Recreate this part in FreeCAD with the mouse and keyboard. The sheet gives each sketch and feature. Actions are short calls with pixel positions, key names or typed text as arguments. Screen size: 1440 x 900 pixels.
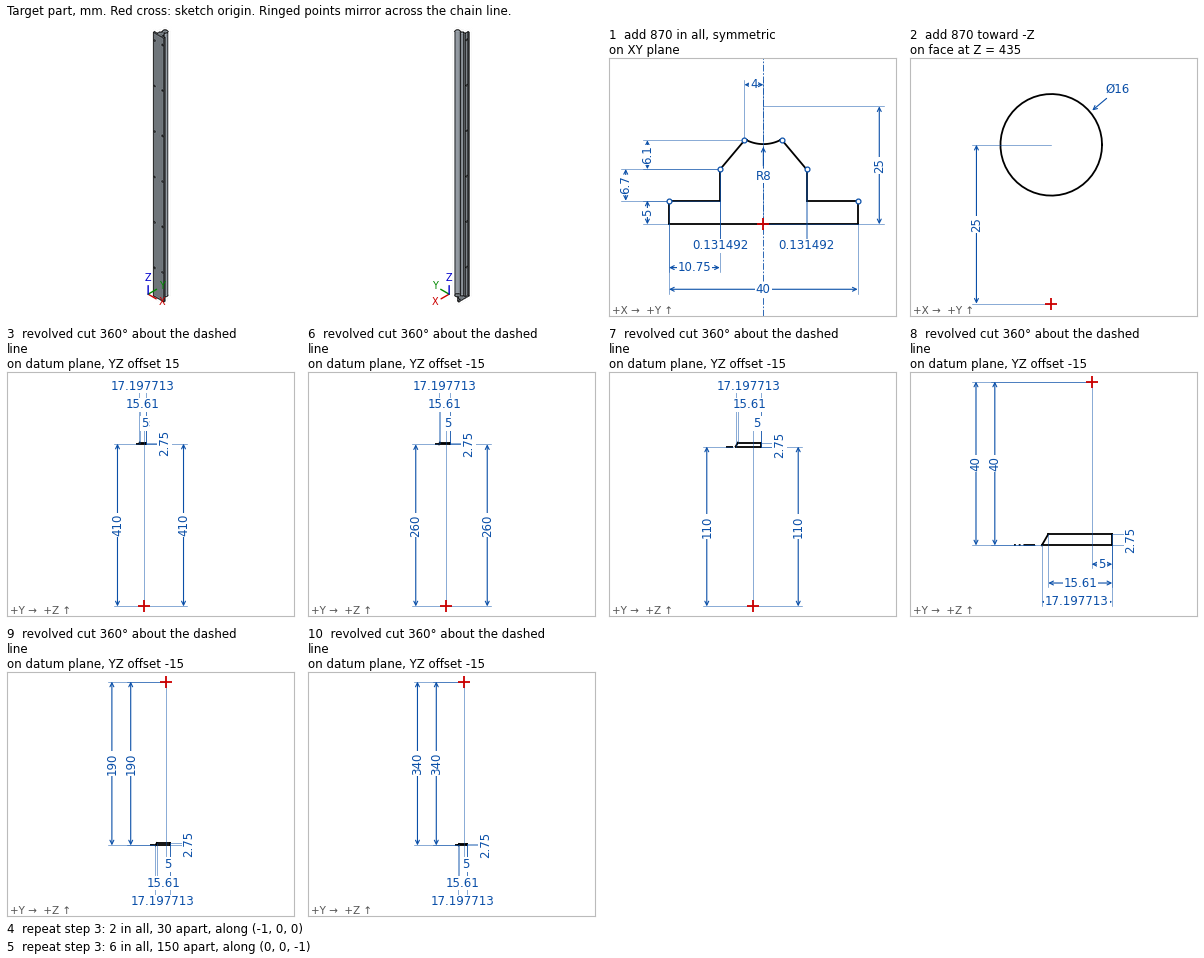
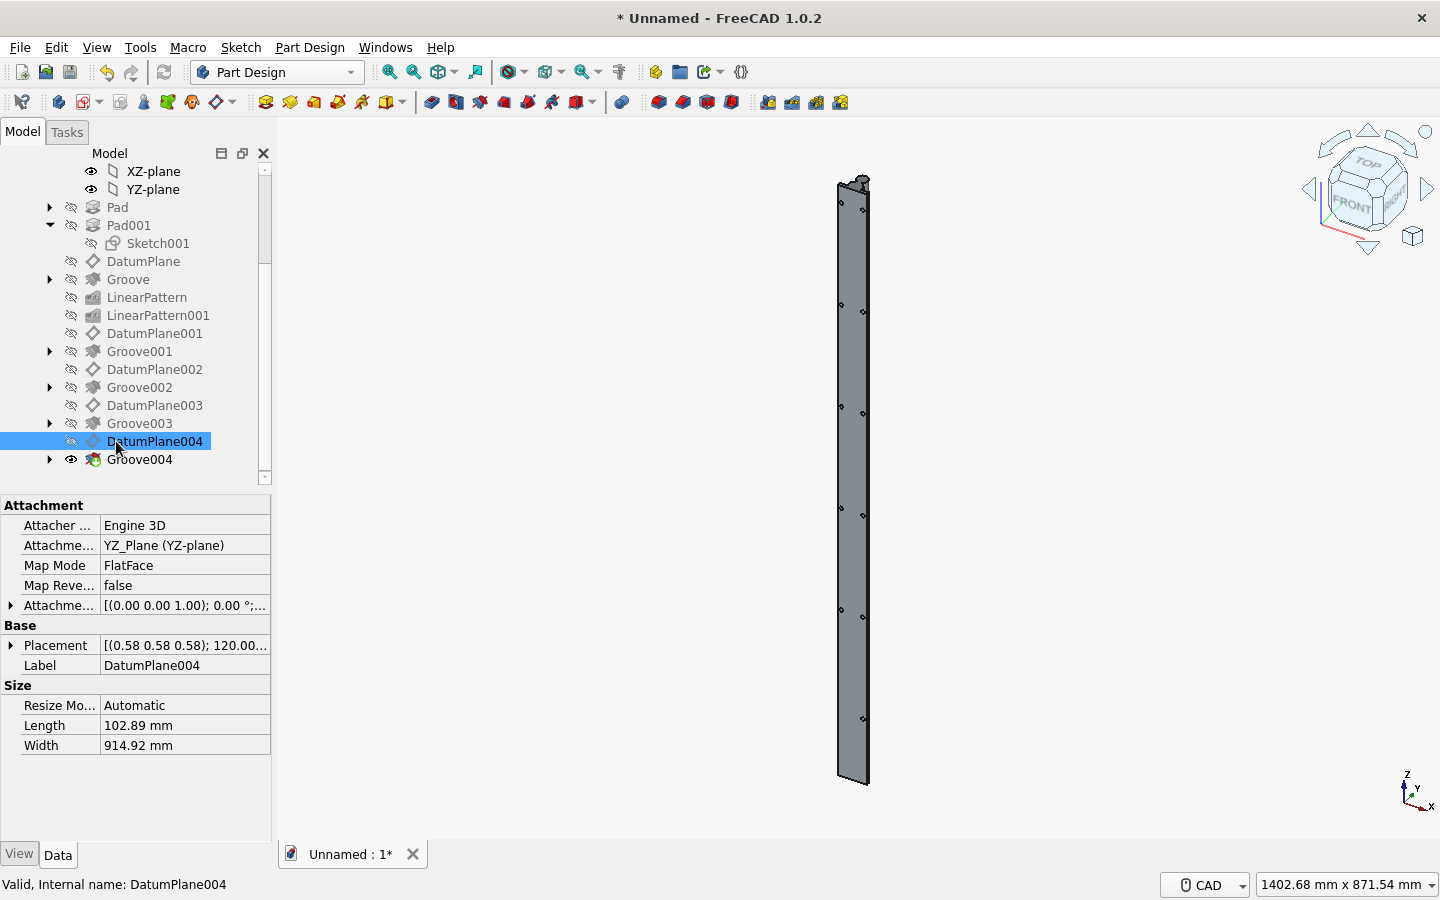
scroll(160, 311, down, 3)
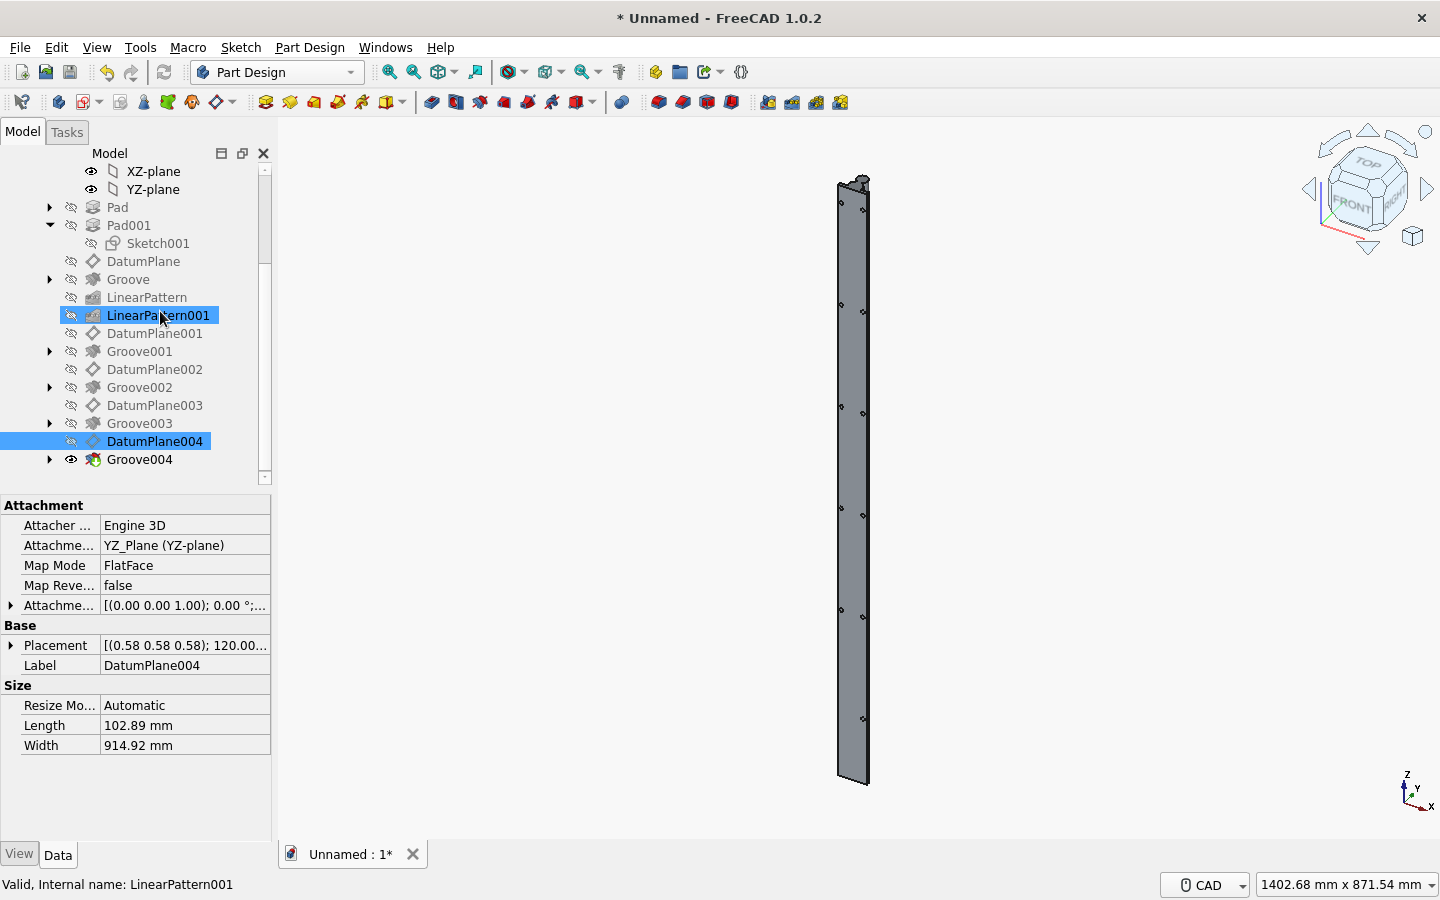
scroll(160, 311, up, 15)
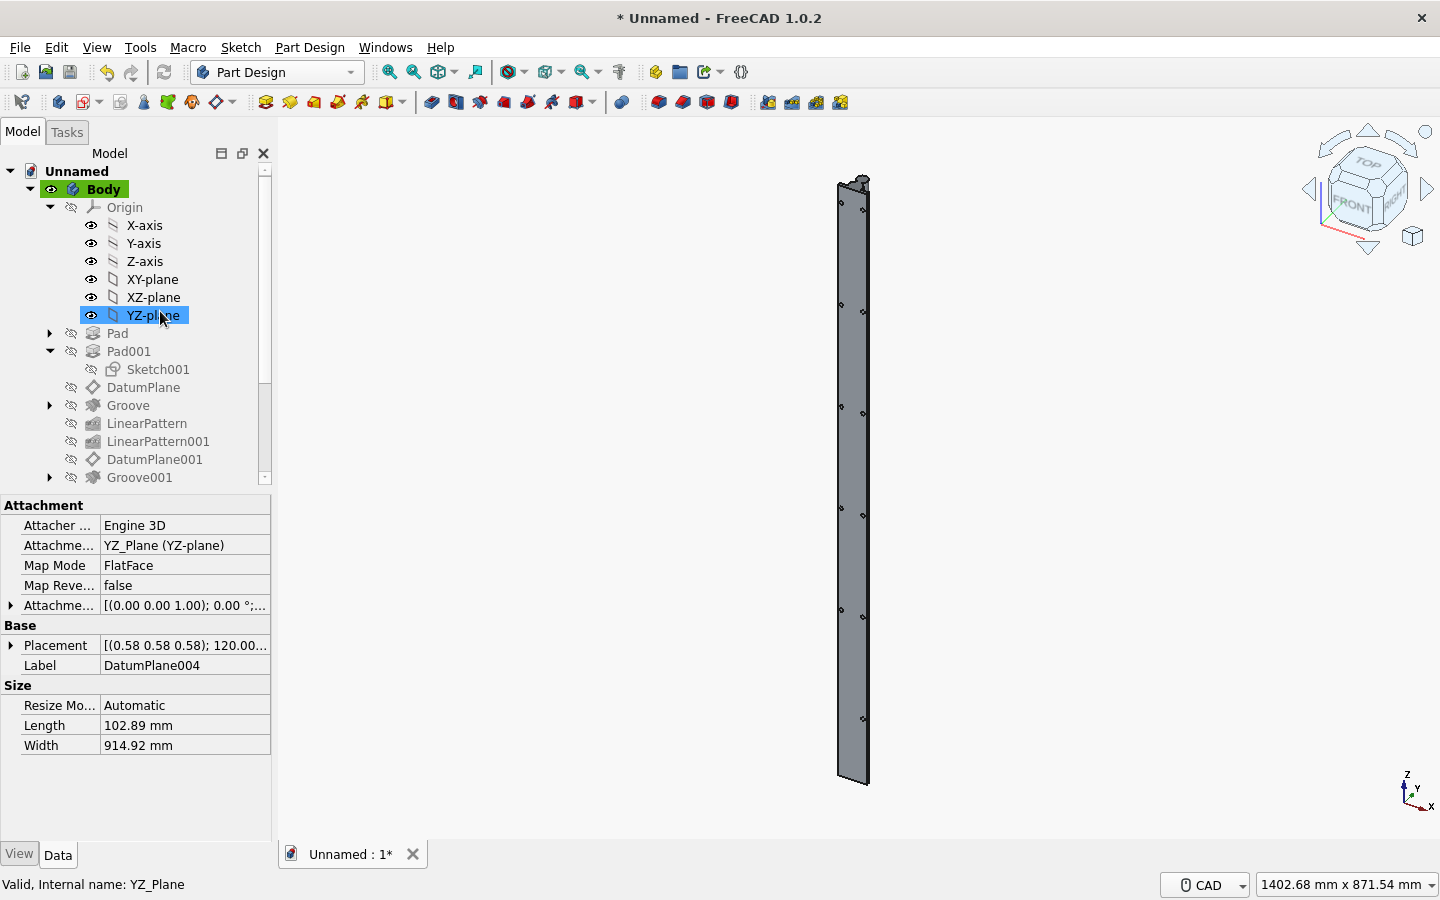
click(136, 315)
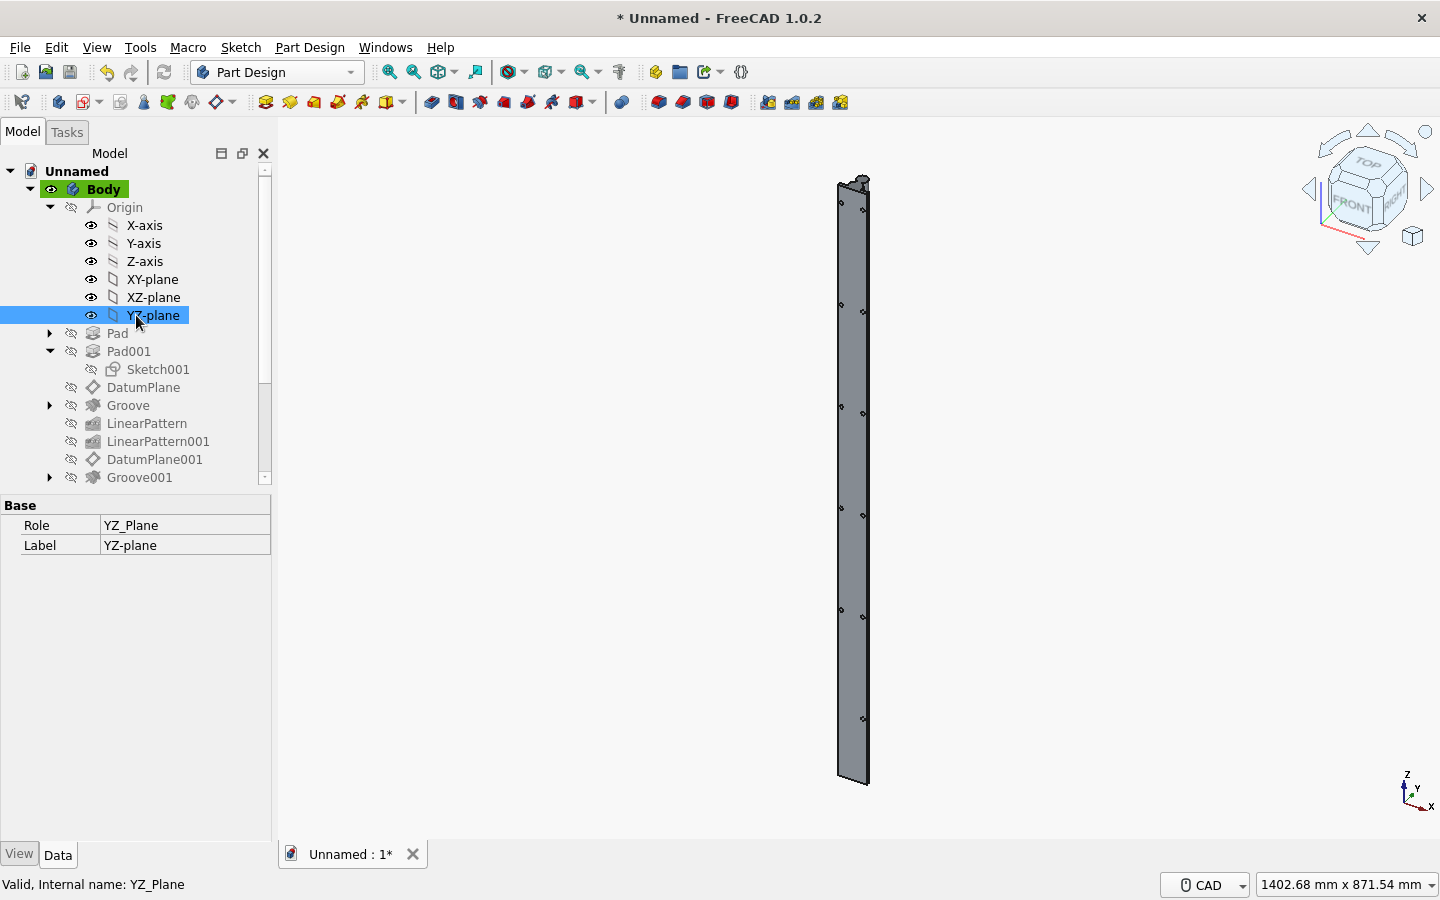
click(216, 102)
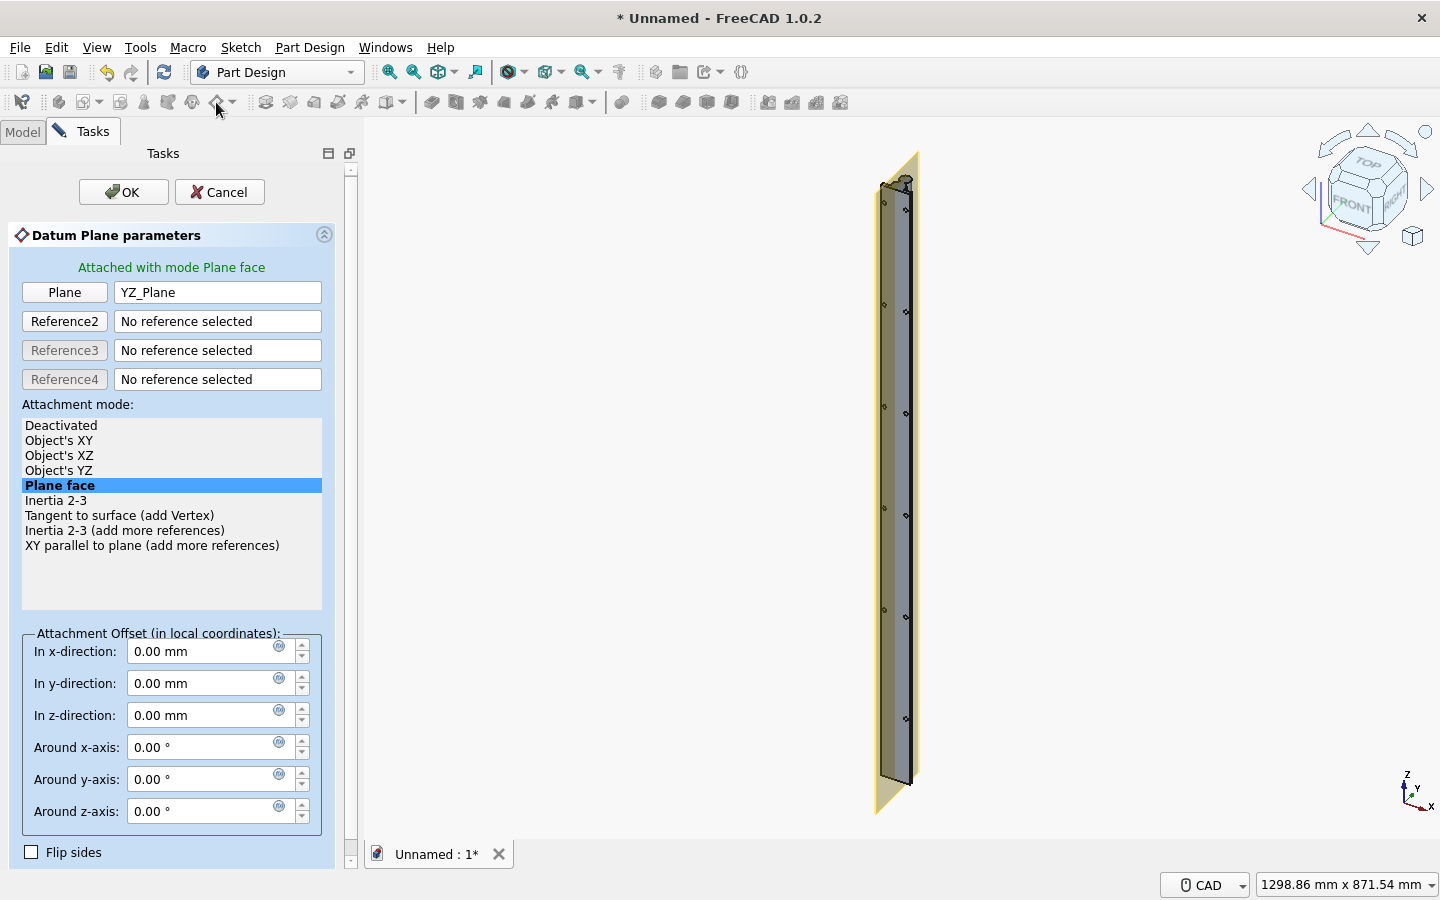
triple_click(210, 715)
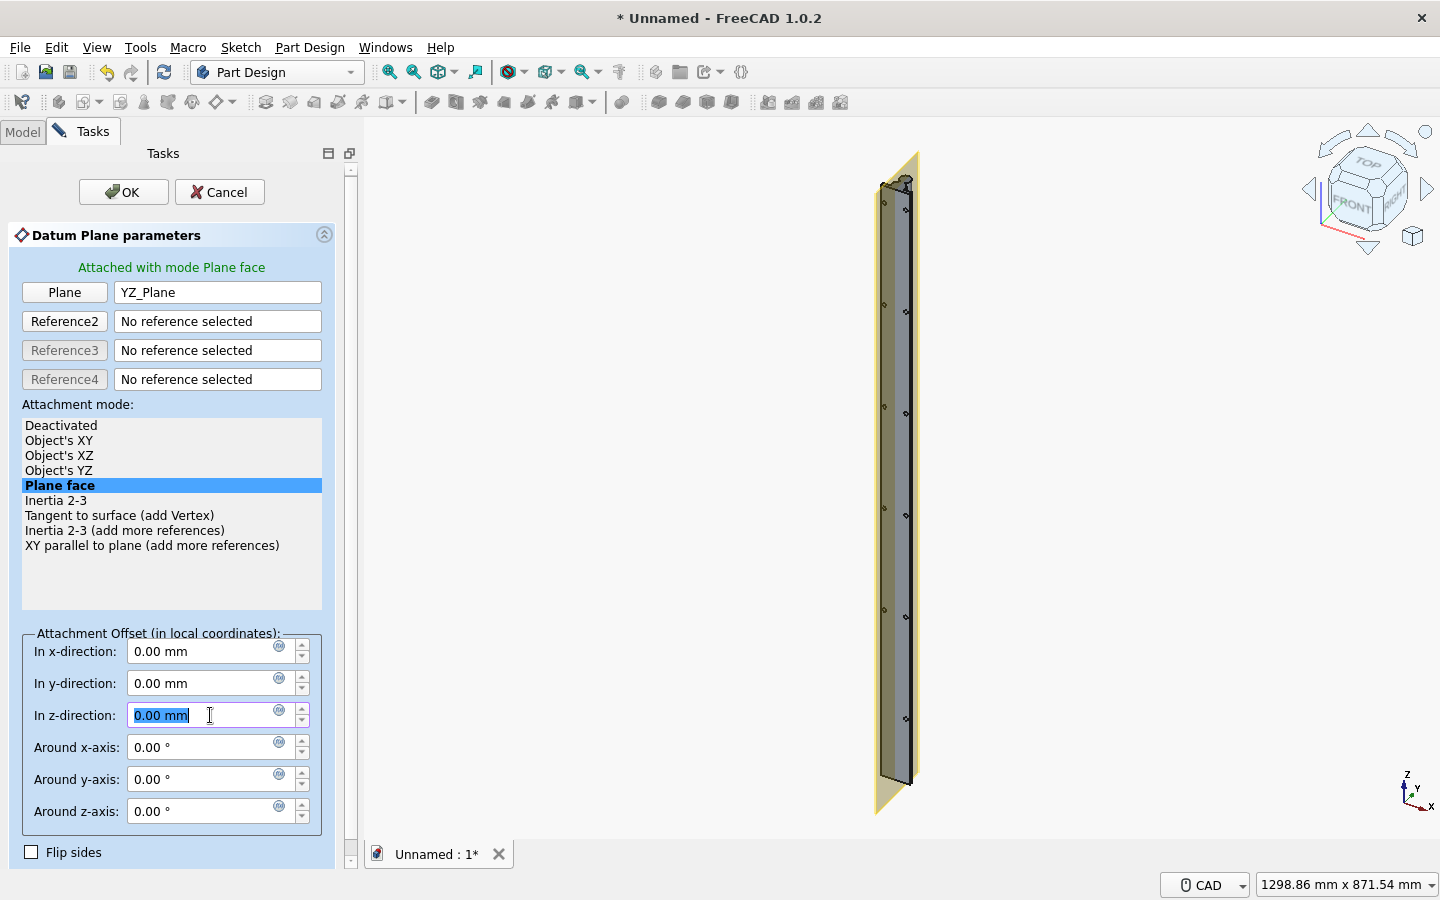
text(-15)
key(Tab)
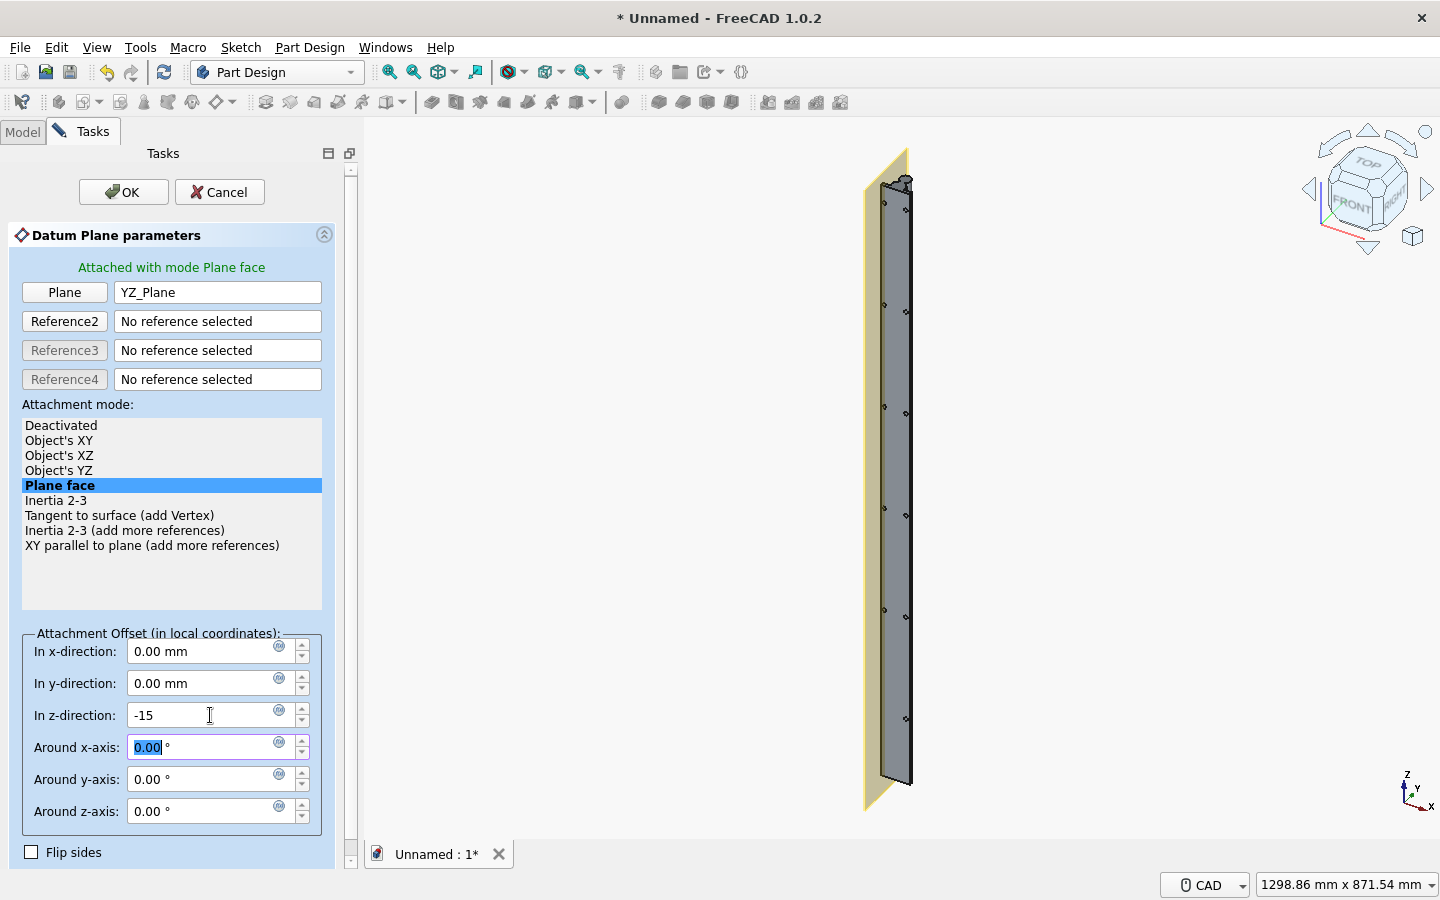
click(124, 192)